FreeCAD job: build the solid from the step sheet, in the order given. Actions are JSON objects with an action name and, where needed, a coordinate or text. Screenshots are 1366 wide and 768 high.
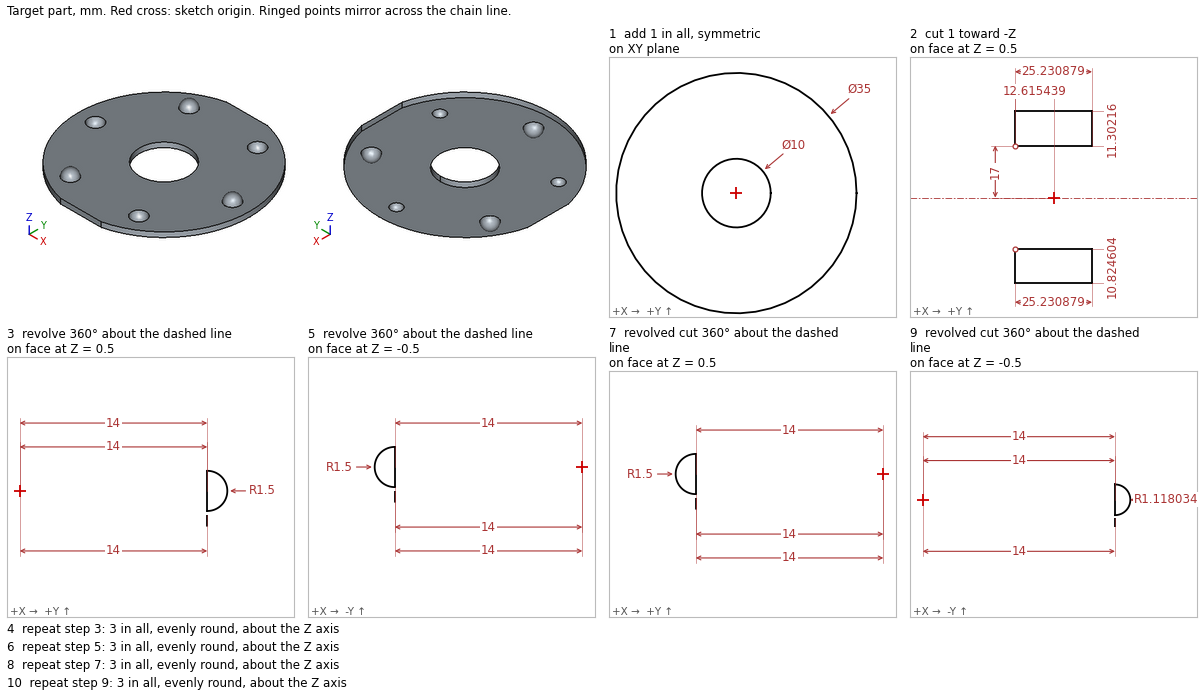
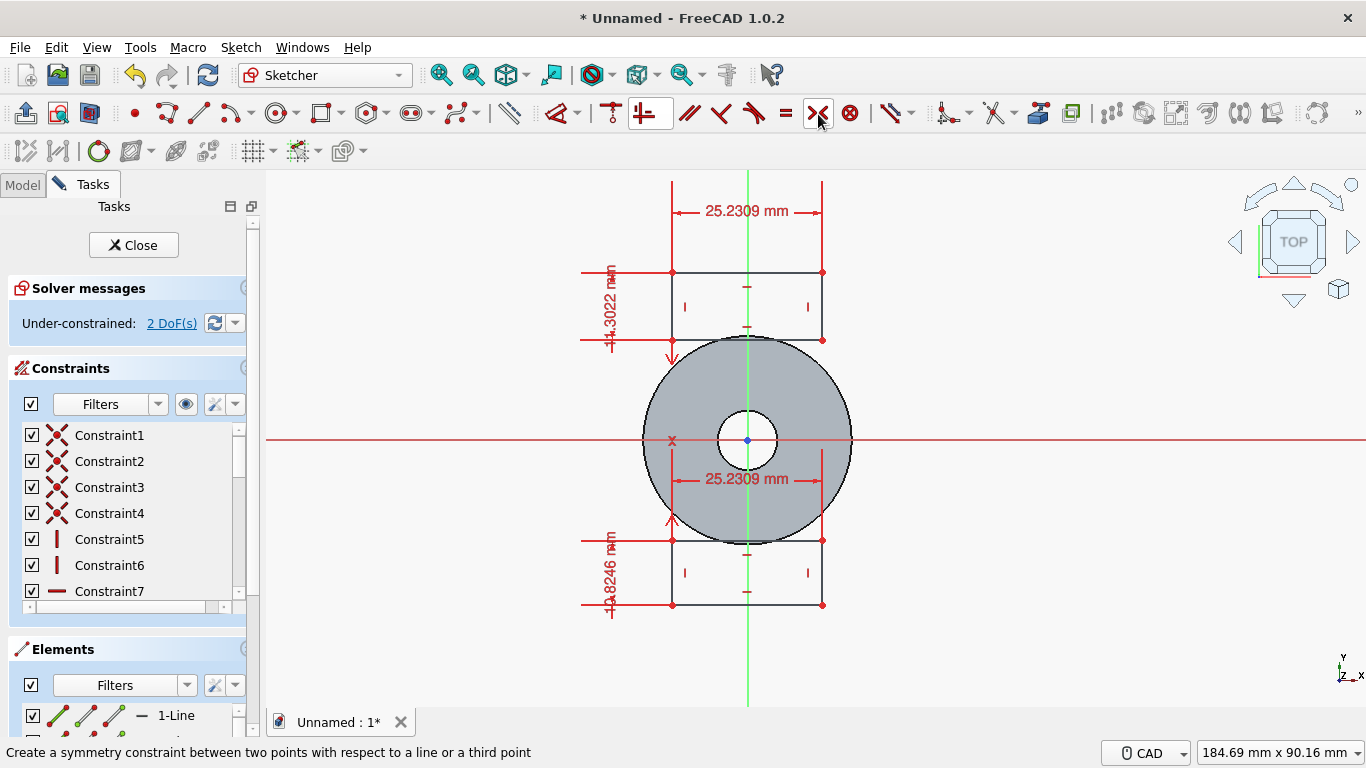
{"action": "left_click", "coordinate": [672, 340]}
{"action": "left_click", "coordinate": [638, 390]}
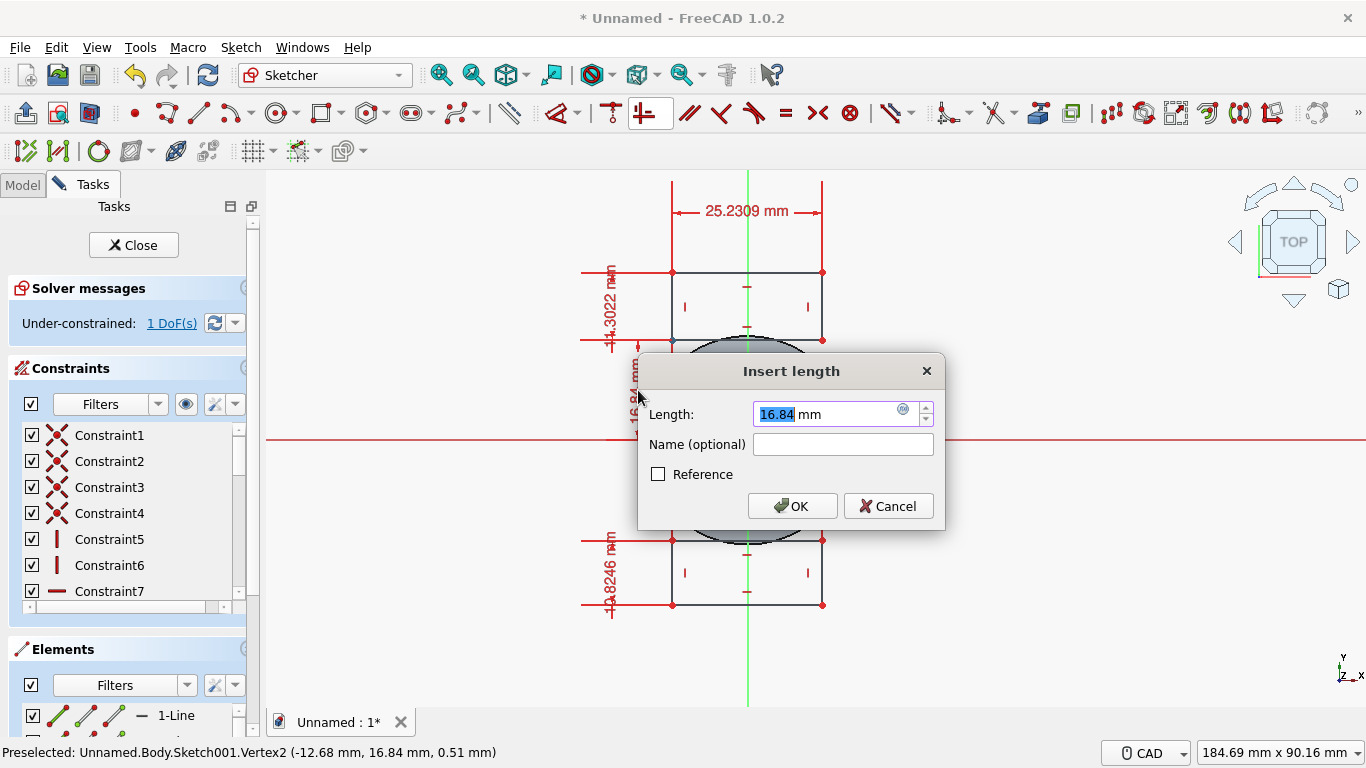
{"action": "type", "text": "17"}
{"action": "key", "text": "Return"}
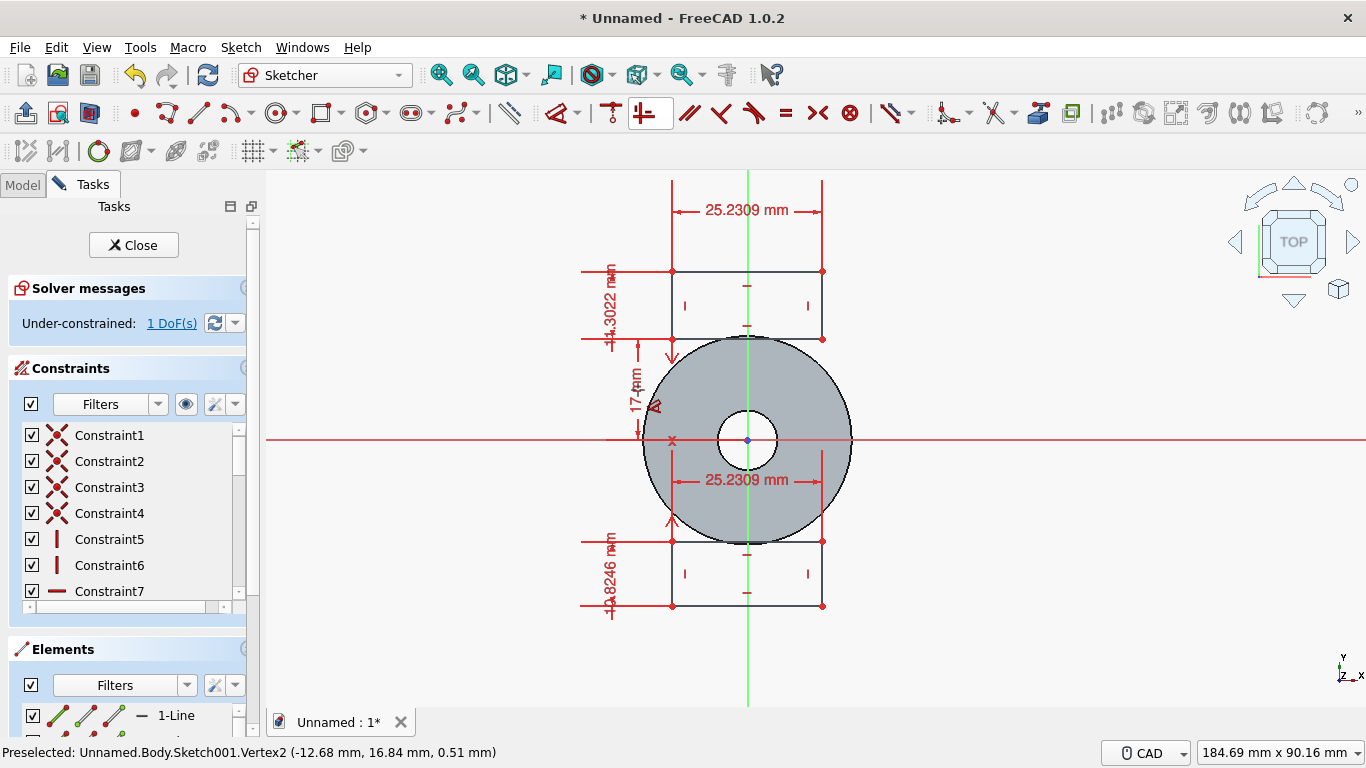
{"action": "left_click", "coordinate": [672, 272]}
{"action": "left_click", "coordinate": [710, 238]}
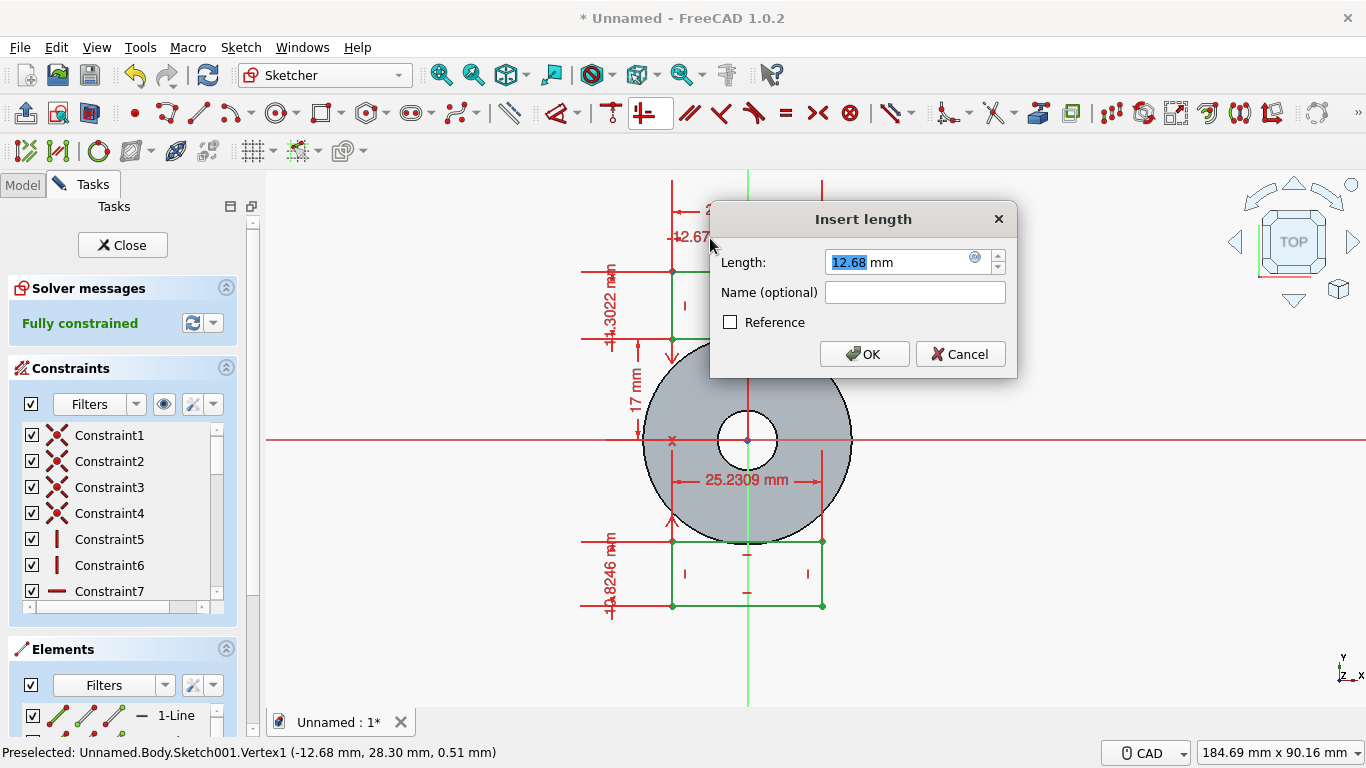
{"action": "type", "text": "12.615439"}
{"action": "key", "text": "Return"}
{"action": "key", "text": "Escape"}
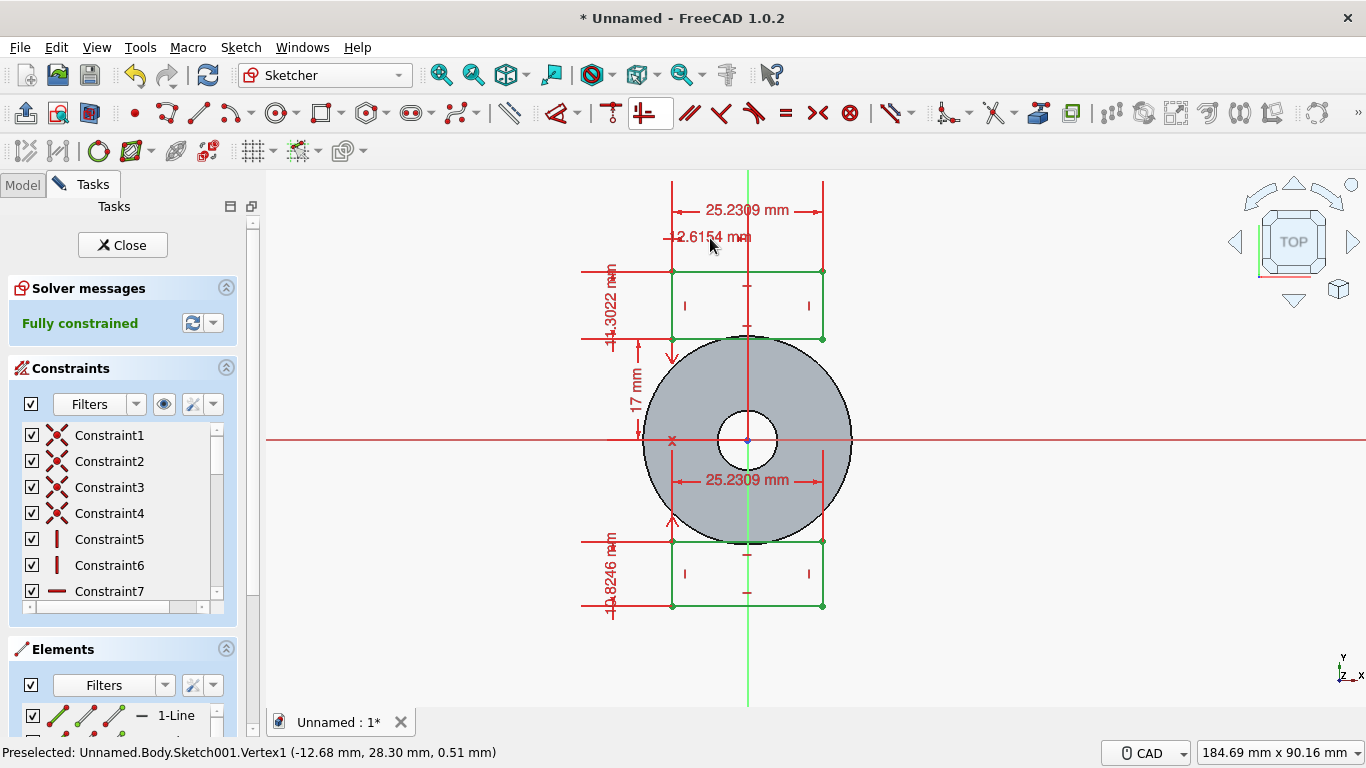
{"action": "left_click", "coordinate": [123, 245]}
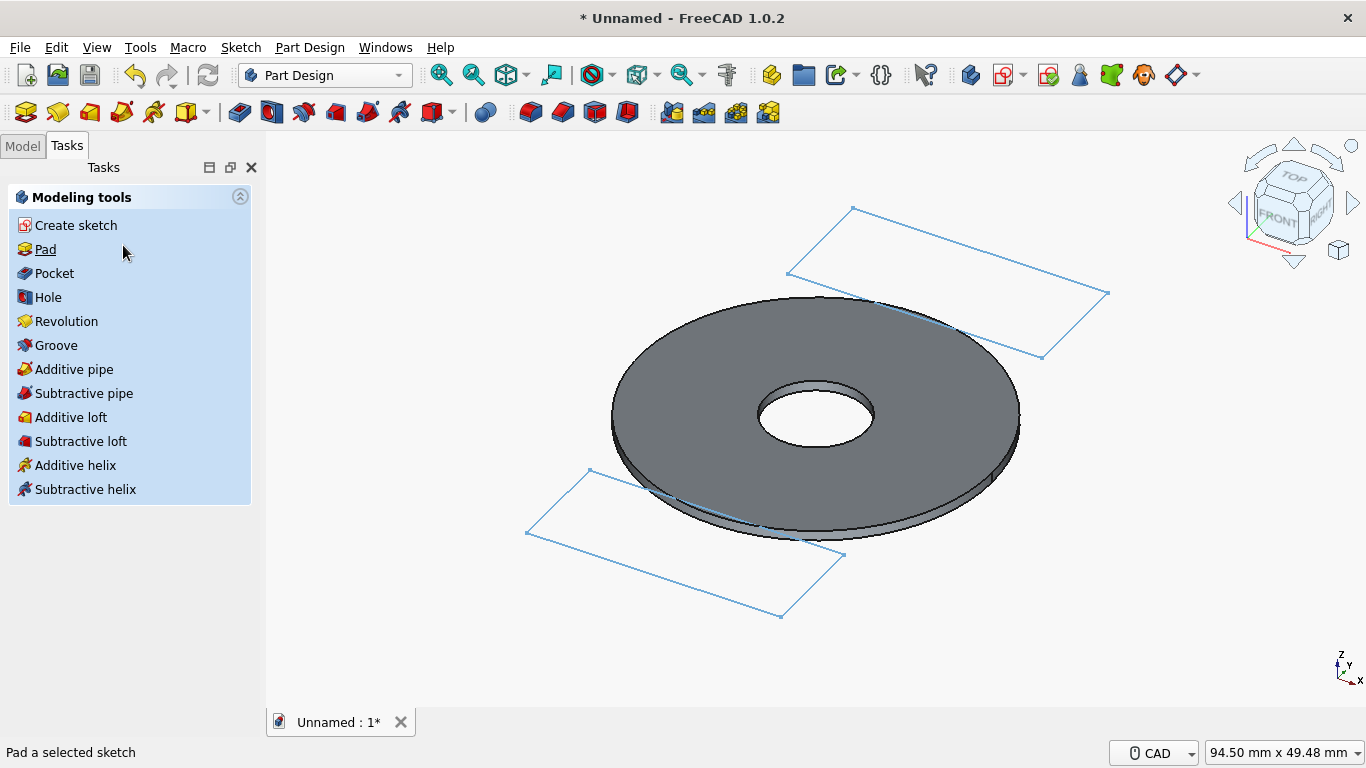
{"action": "left_click", "coordinate": [240, 112]}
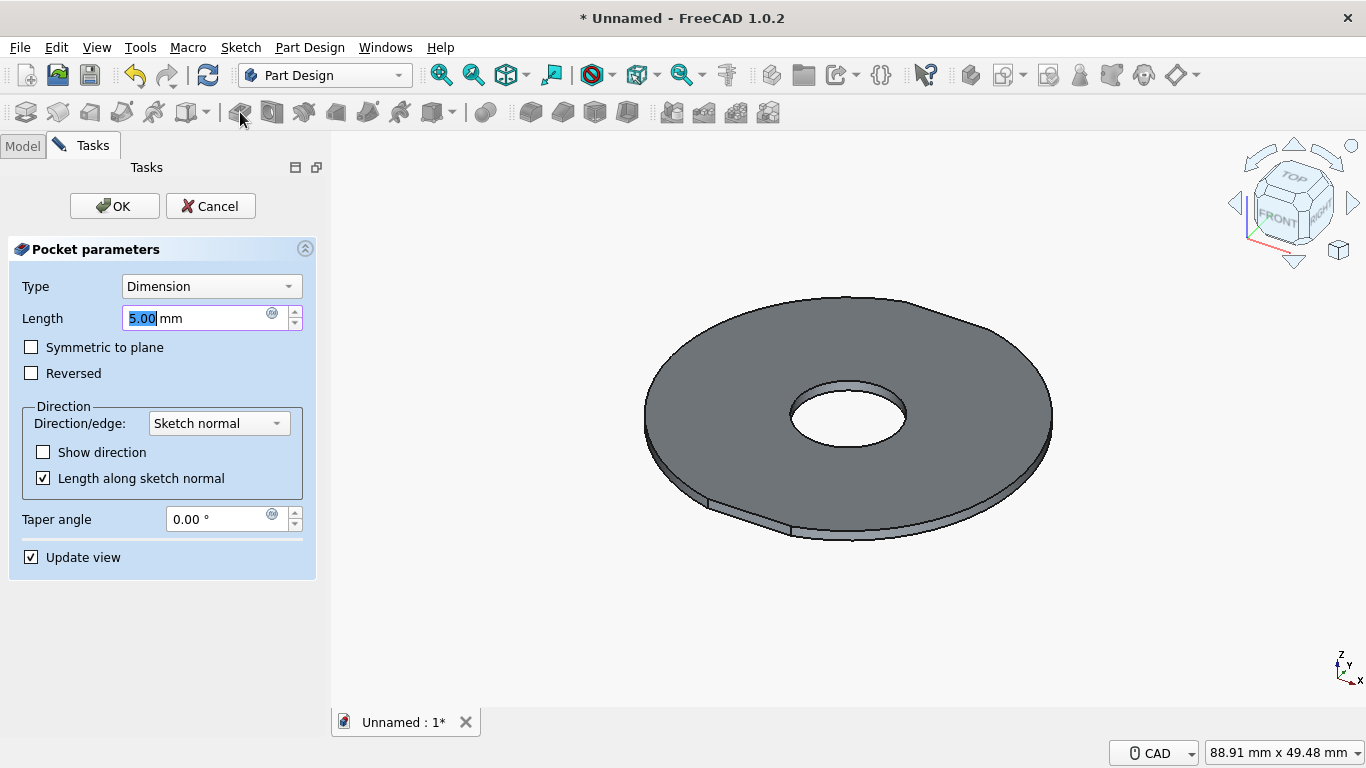
{"action": "type", "text": "1"}
{"action": "key", "text": "Tab"}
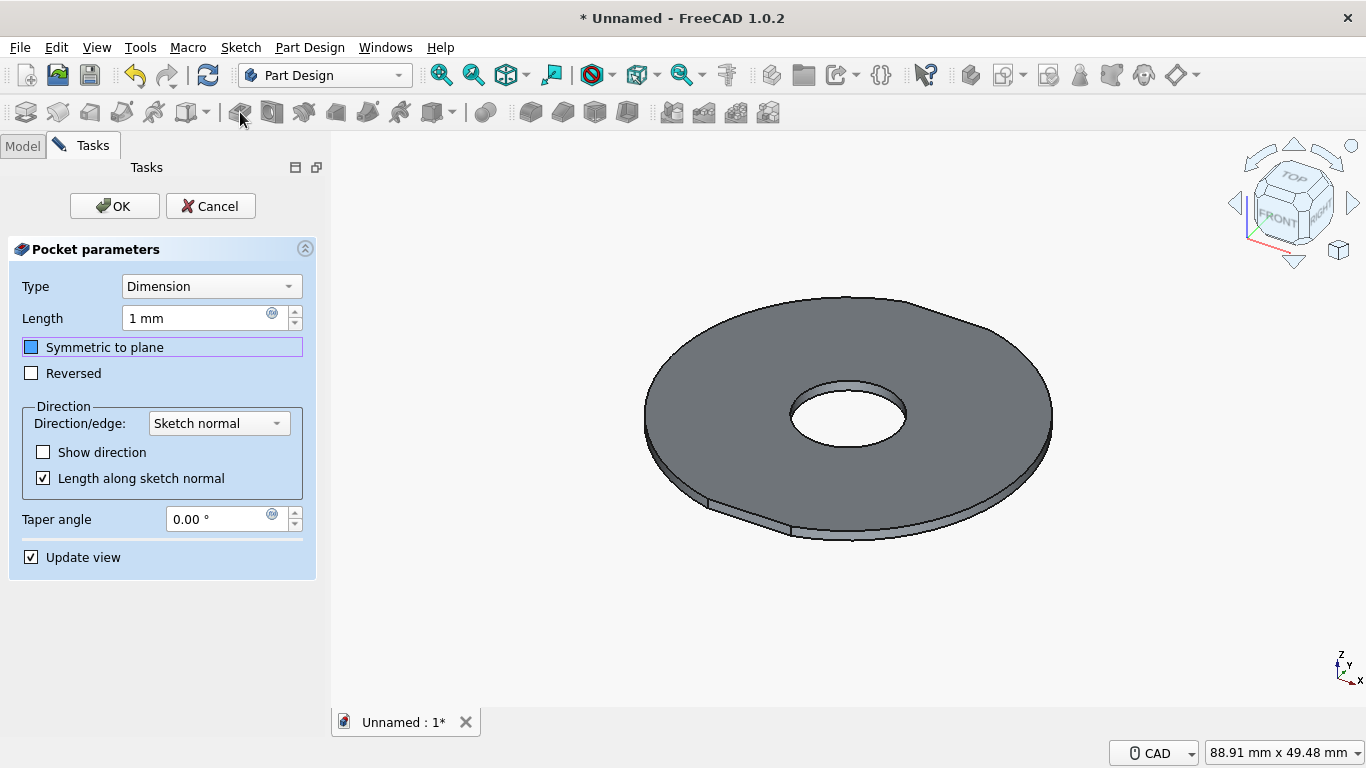
{"action": "left_click", "coordinate": [115, 206]}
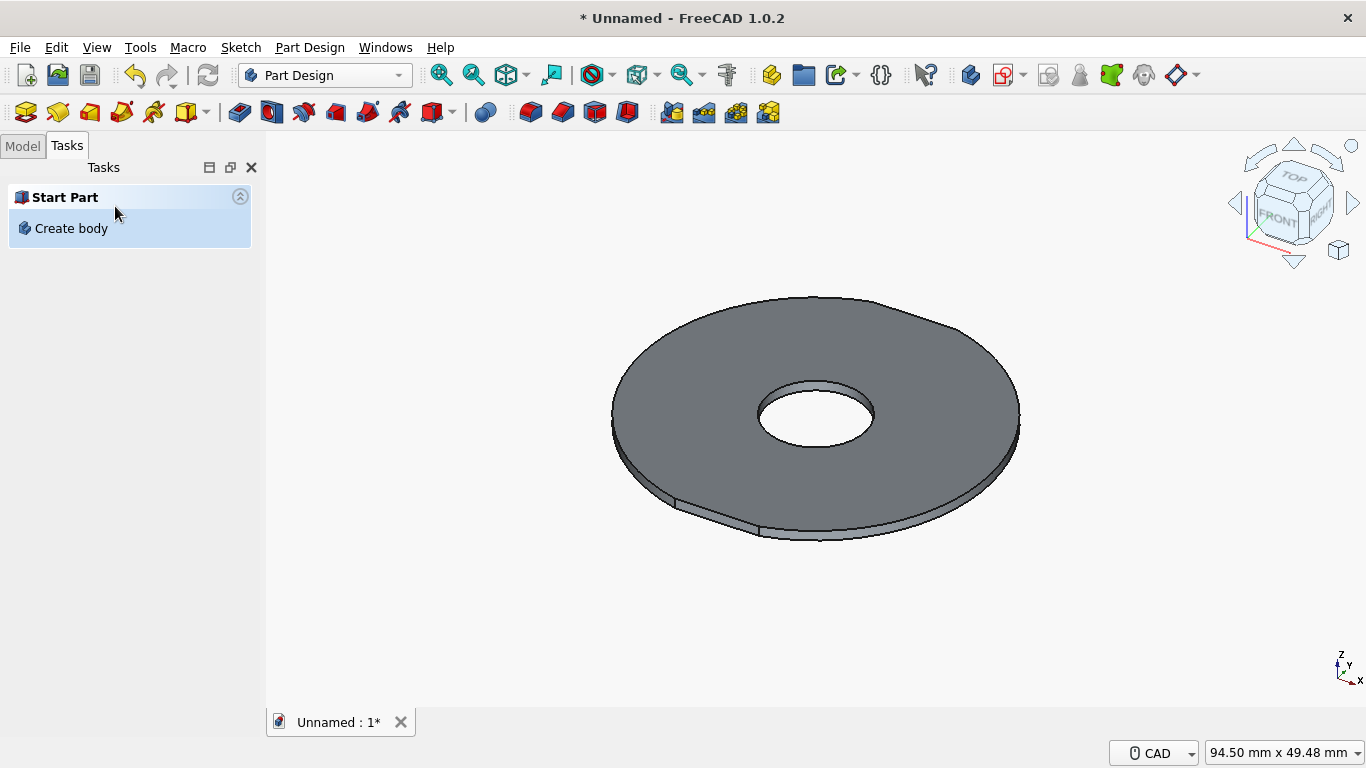
{"action": "left_click", "coordinate": [888, 475]}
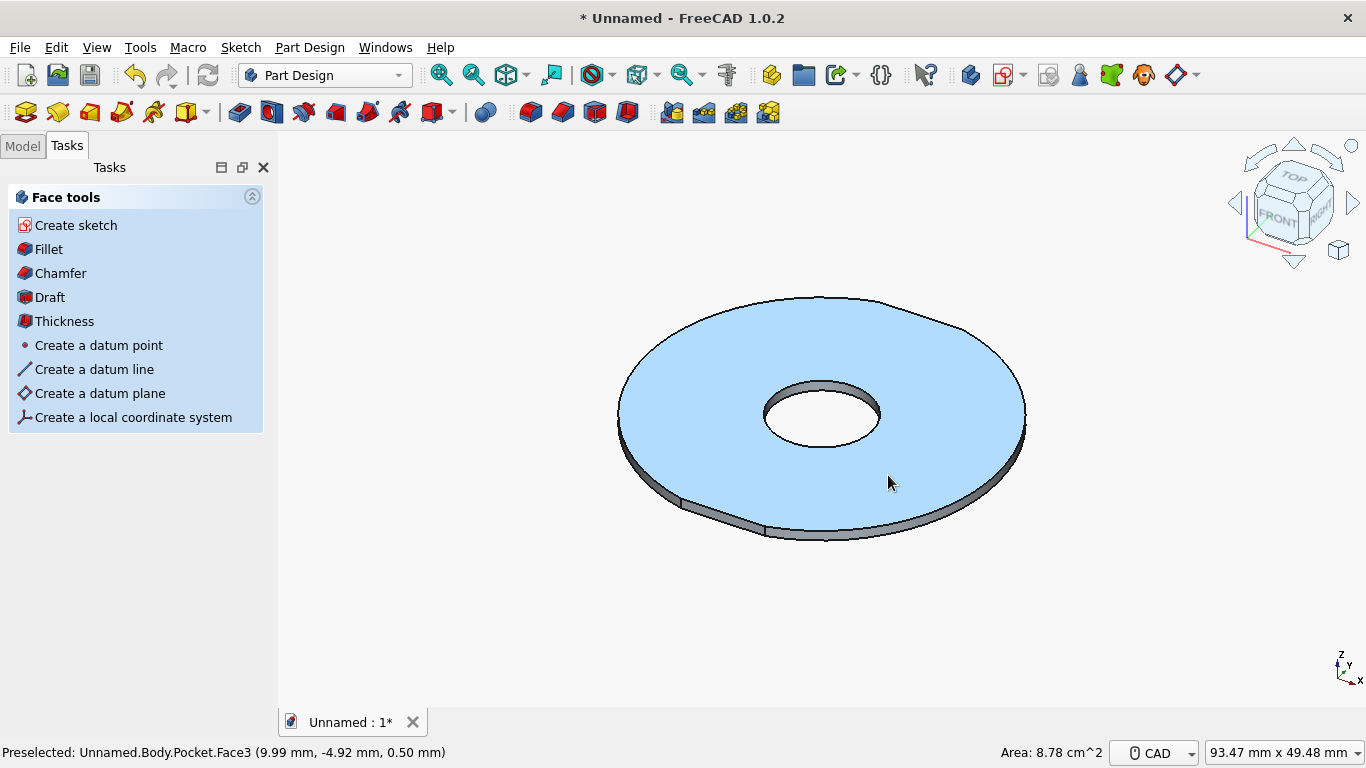
{"action": "left_click", "coordinate": [1004, 76]}